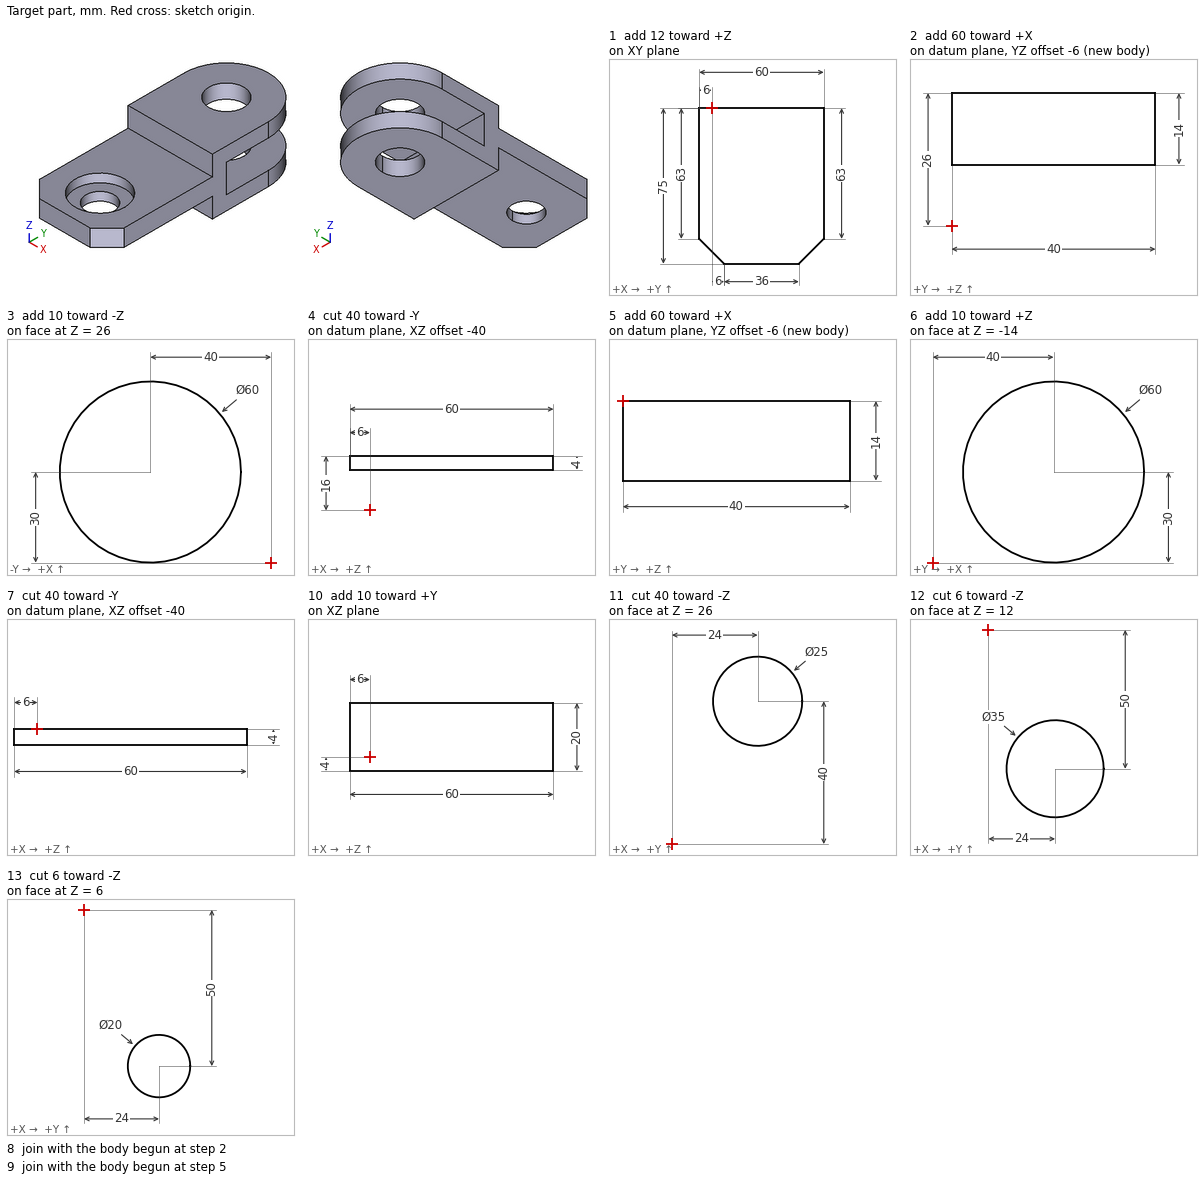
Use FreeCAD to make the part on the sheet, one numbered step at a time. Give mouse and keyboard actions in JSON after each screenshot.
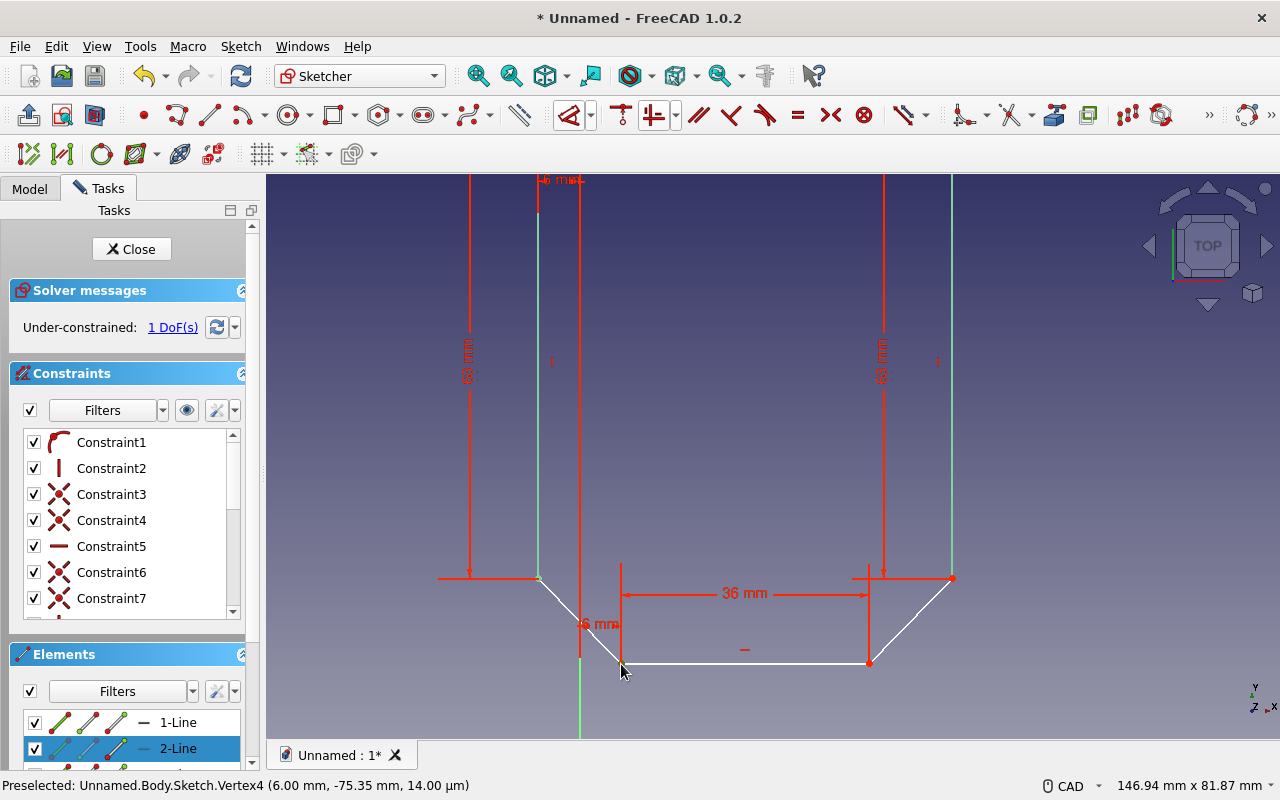
{"action": "key", "text": "i"}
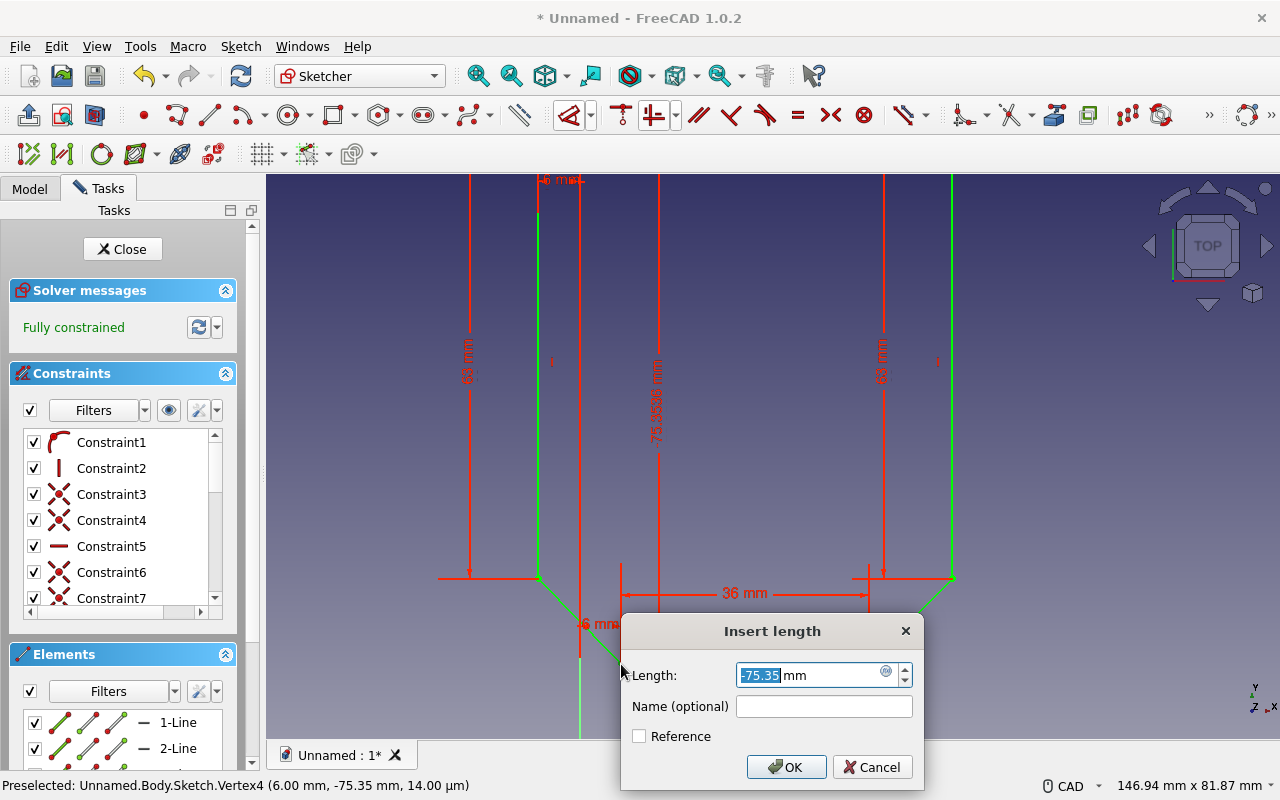
{"action": "type", "text": "-75"}
{"action": "key", "text": "Return"}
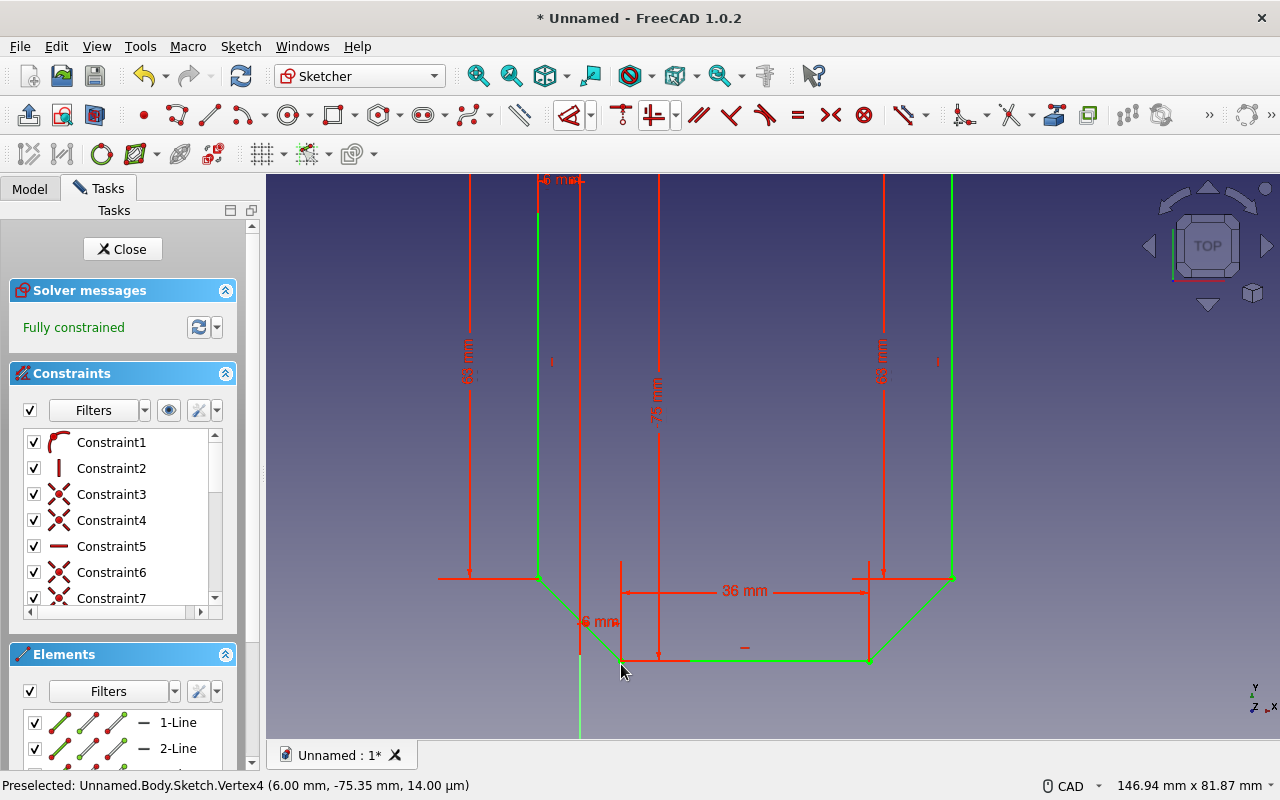
{"action": "left_click", "coordinate": [123, 249]}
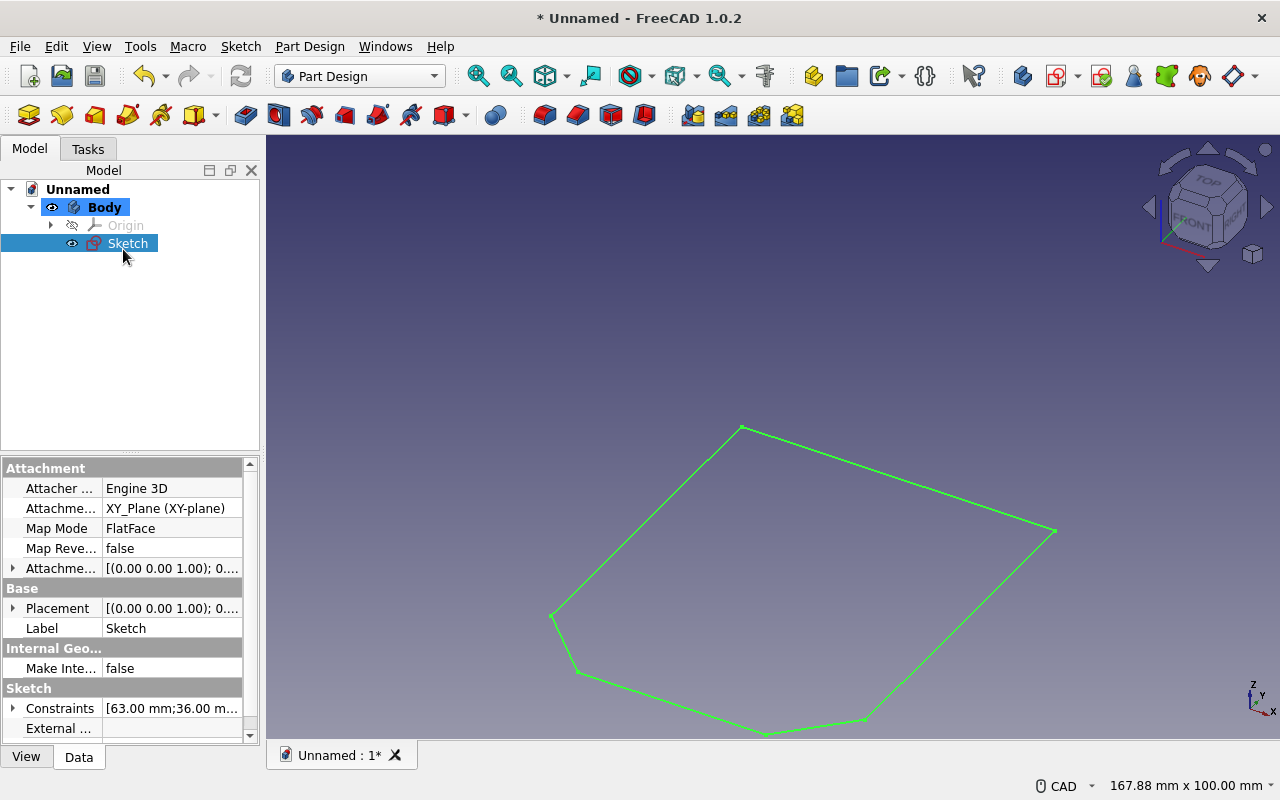
{"action": "left_click", "coordinate": [29, 116]}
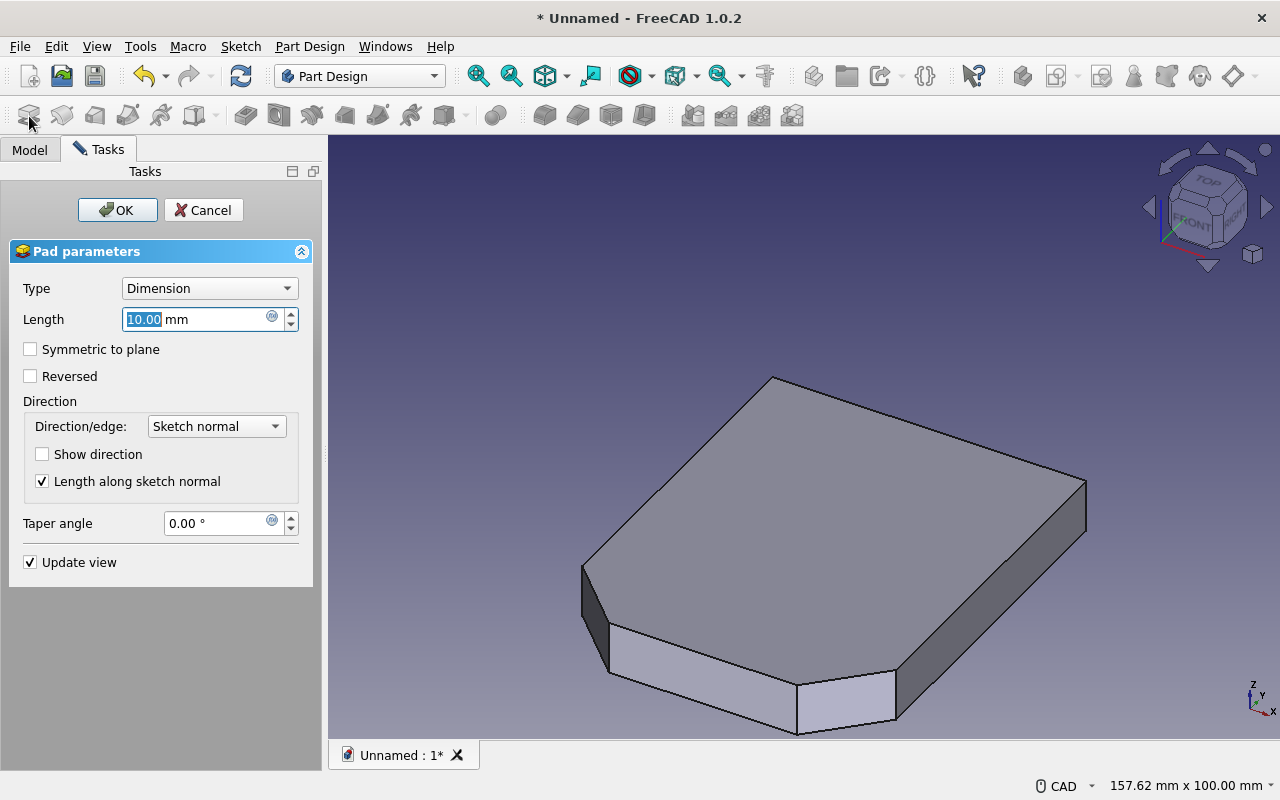
{"action": "type", "text": "12"}
{"action": "key", "text": "Tab"}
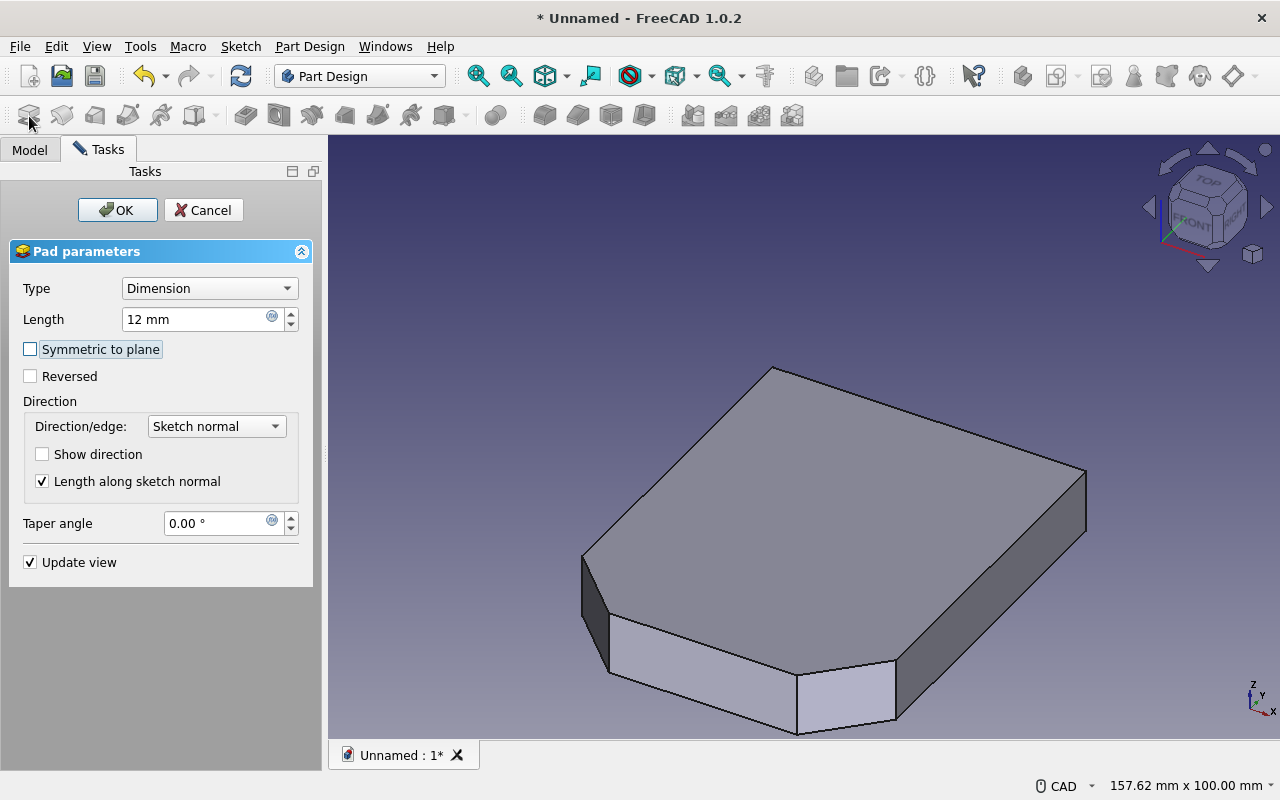
{"action": "left_click", "coordinate": [118, 210]}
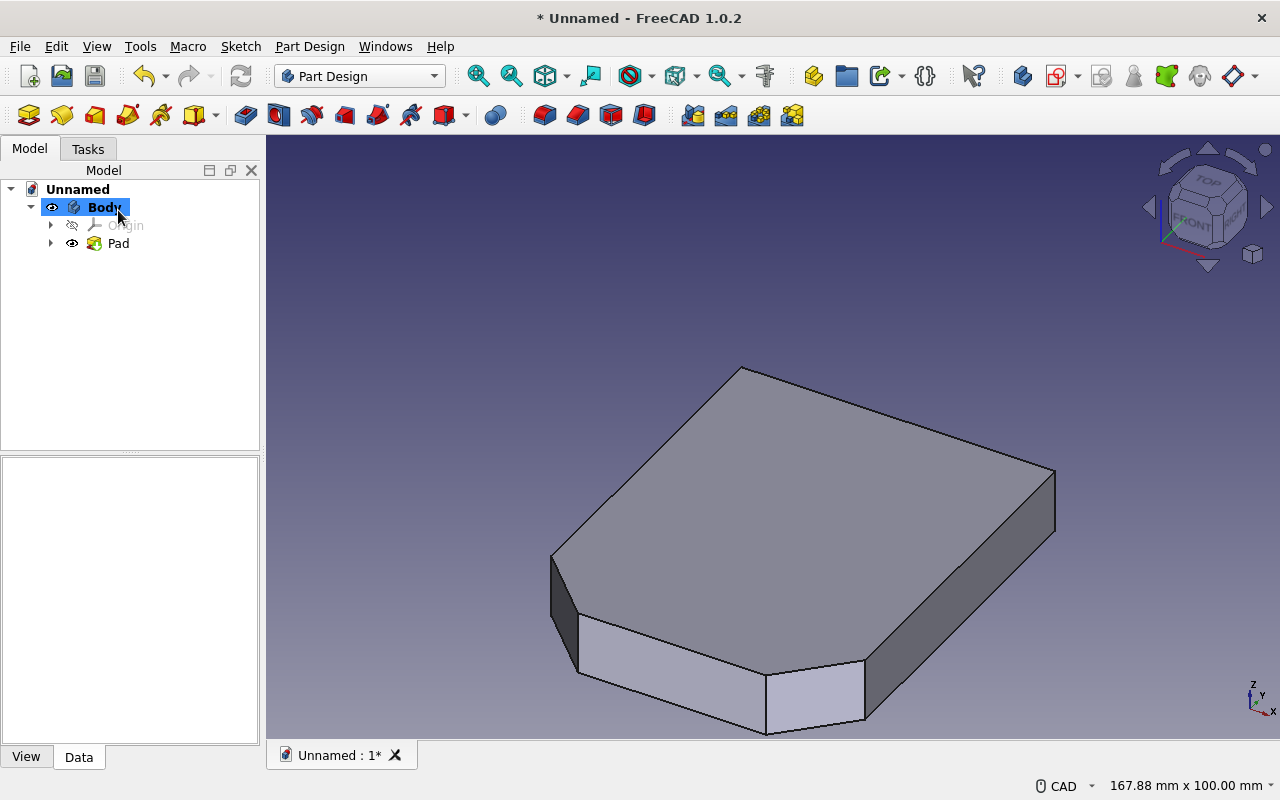
{"action": "left_click", "coordinate": [479, 76]}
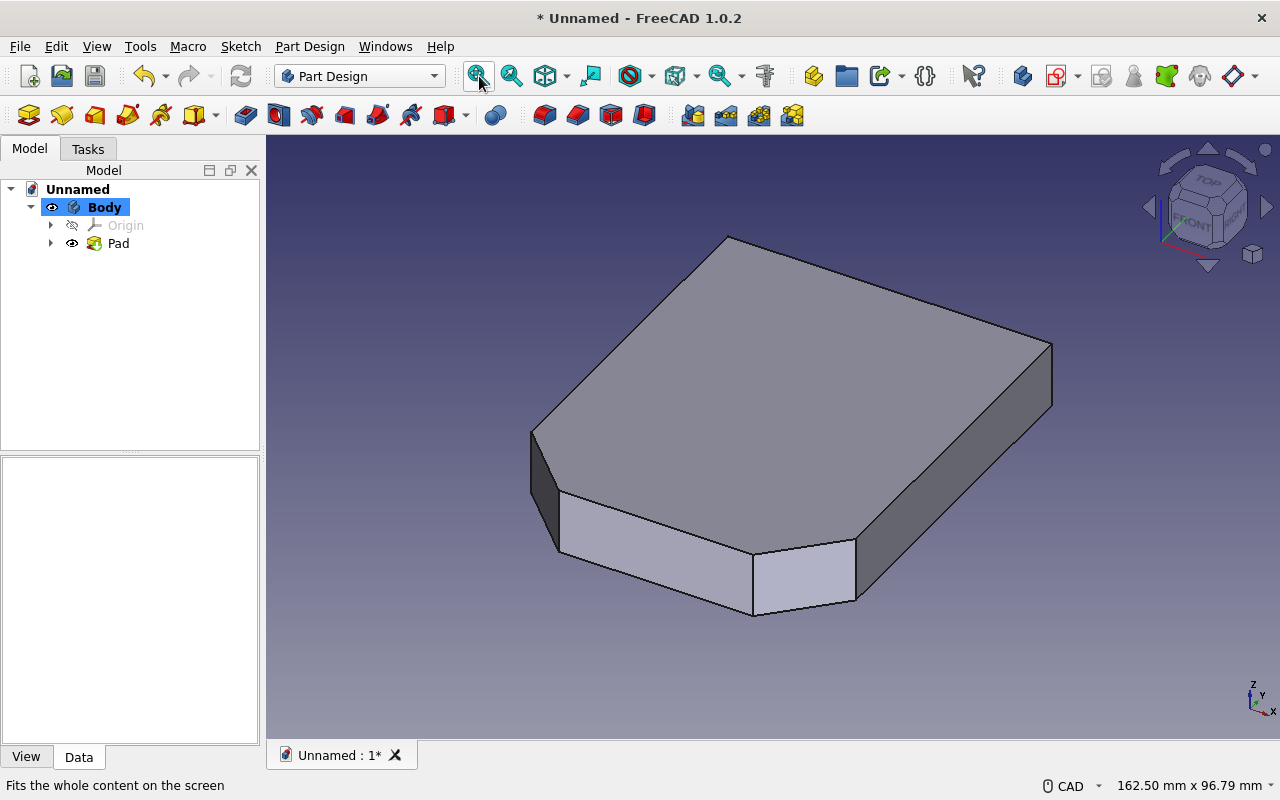
{"action": "left_click", "coordinate": [1023, 76]}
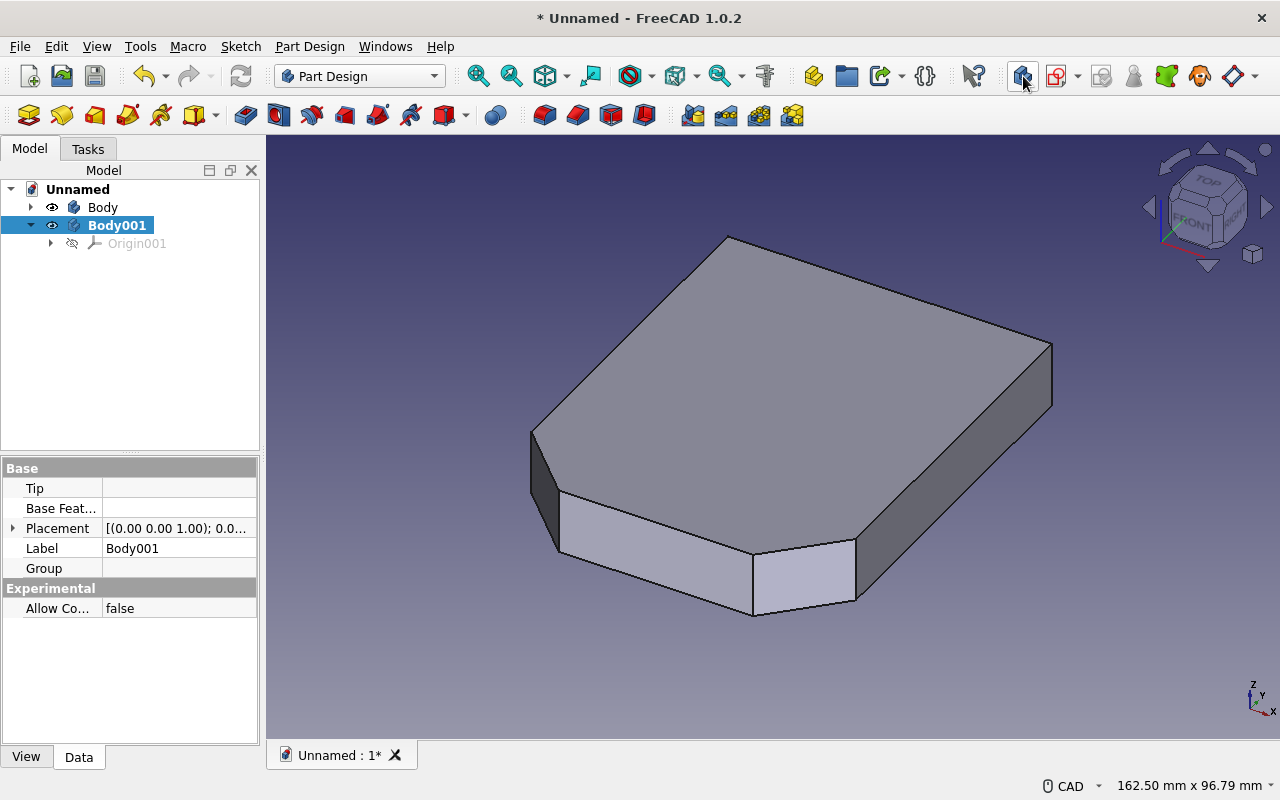
{"action": "left_click", "coordinate": [51, 243]}